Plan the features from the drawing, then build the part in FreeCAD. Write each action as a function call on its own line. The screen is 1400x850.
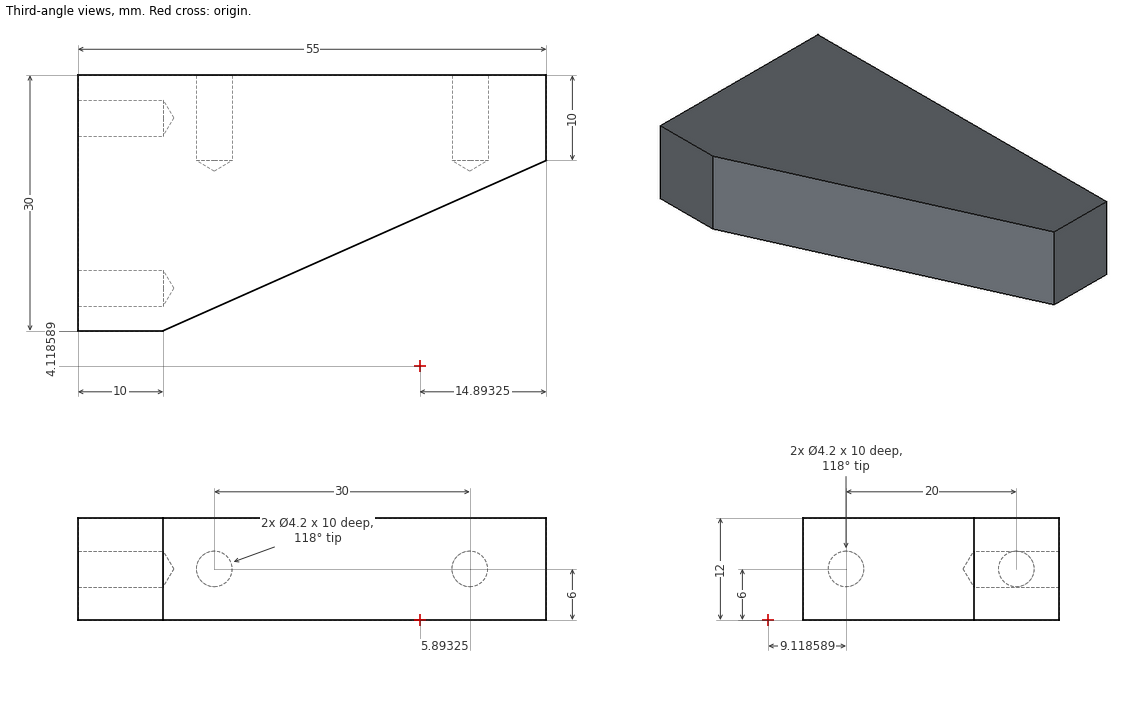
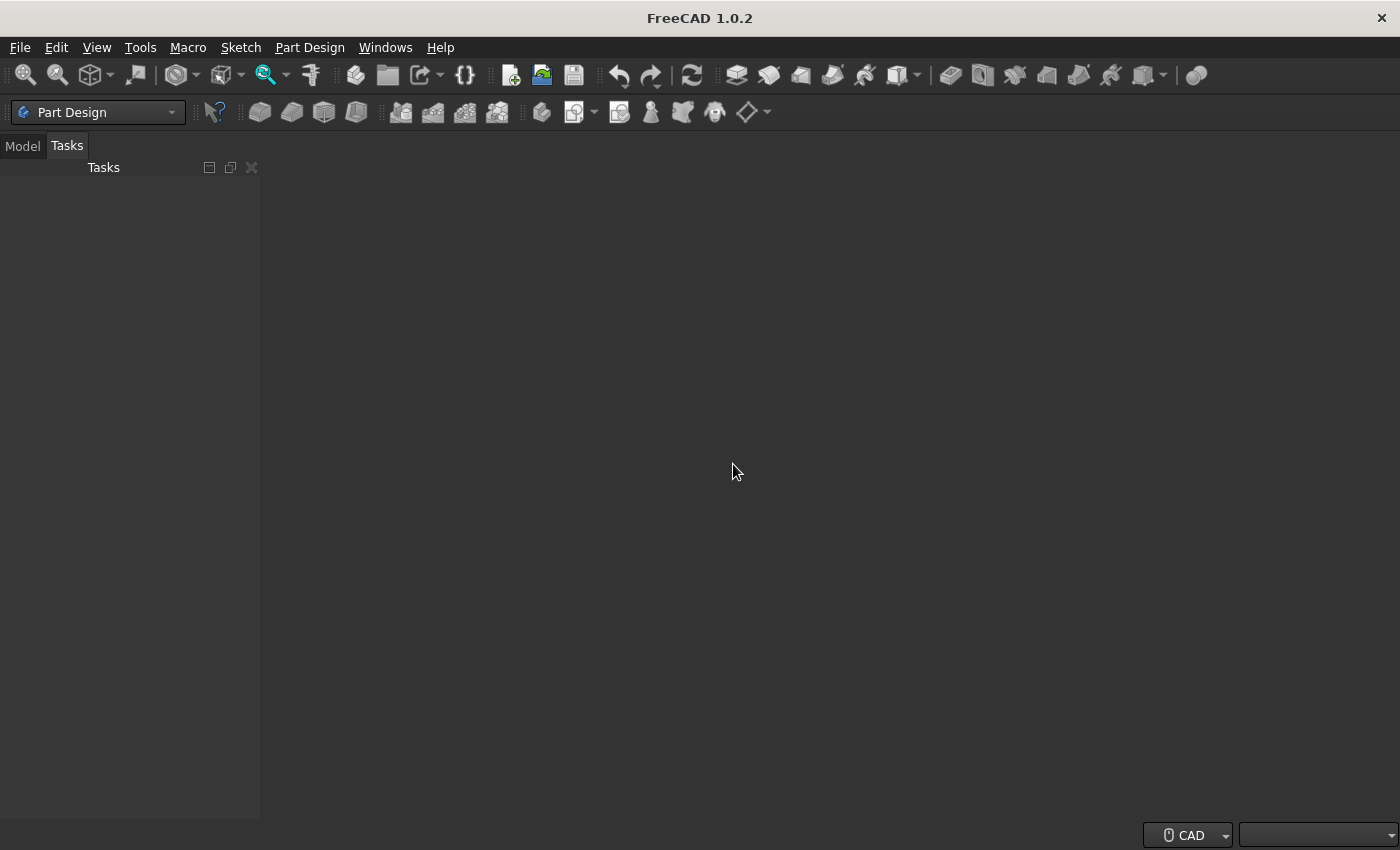
click(510, 76)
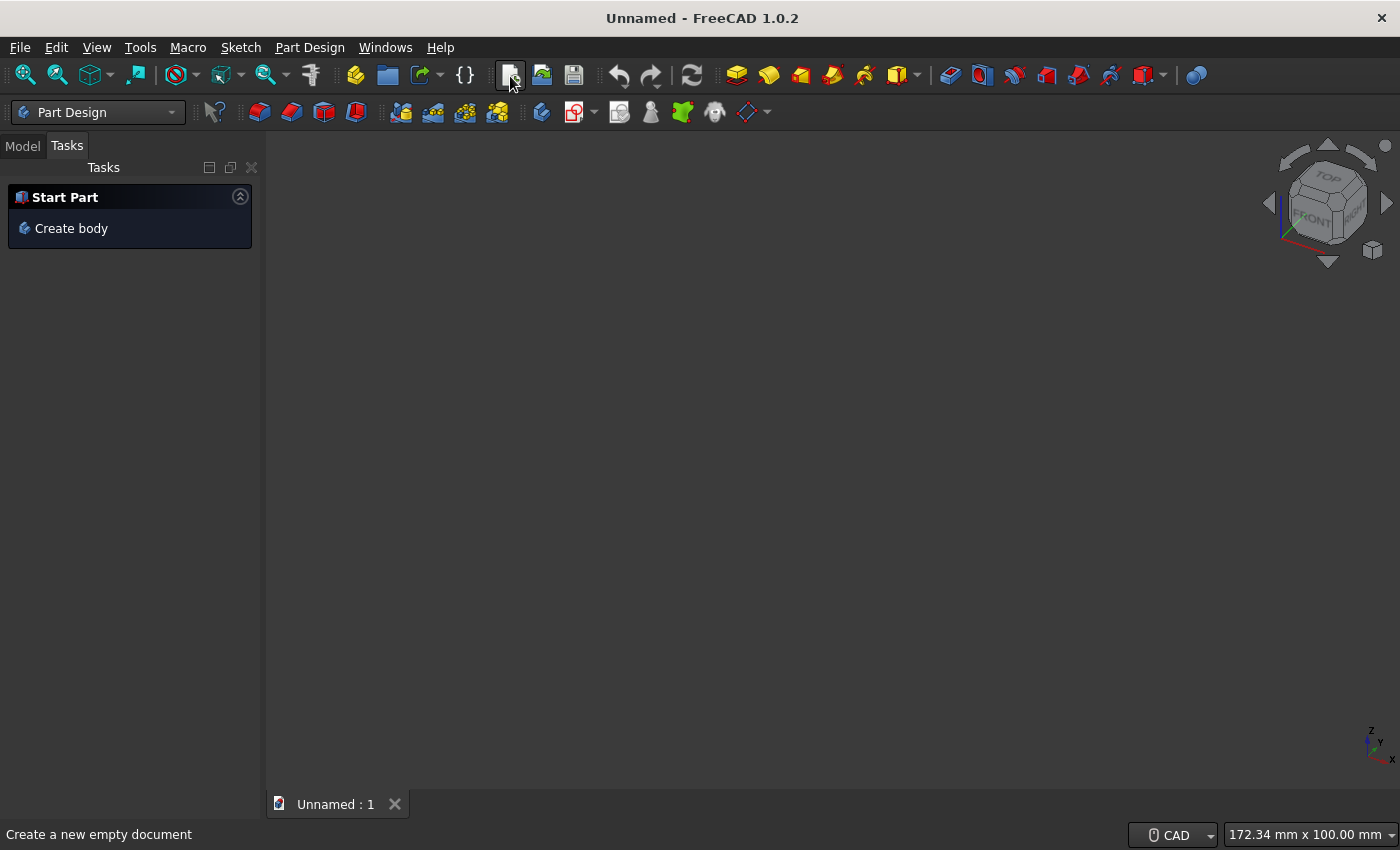
click(574, 112)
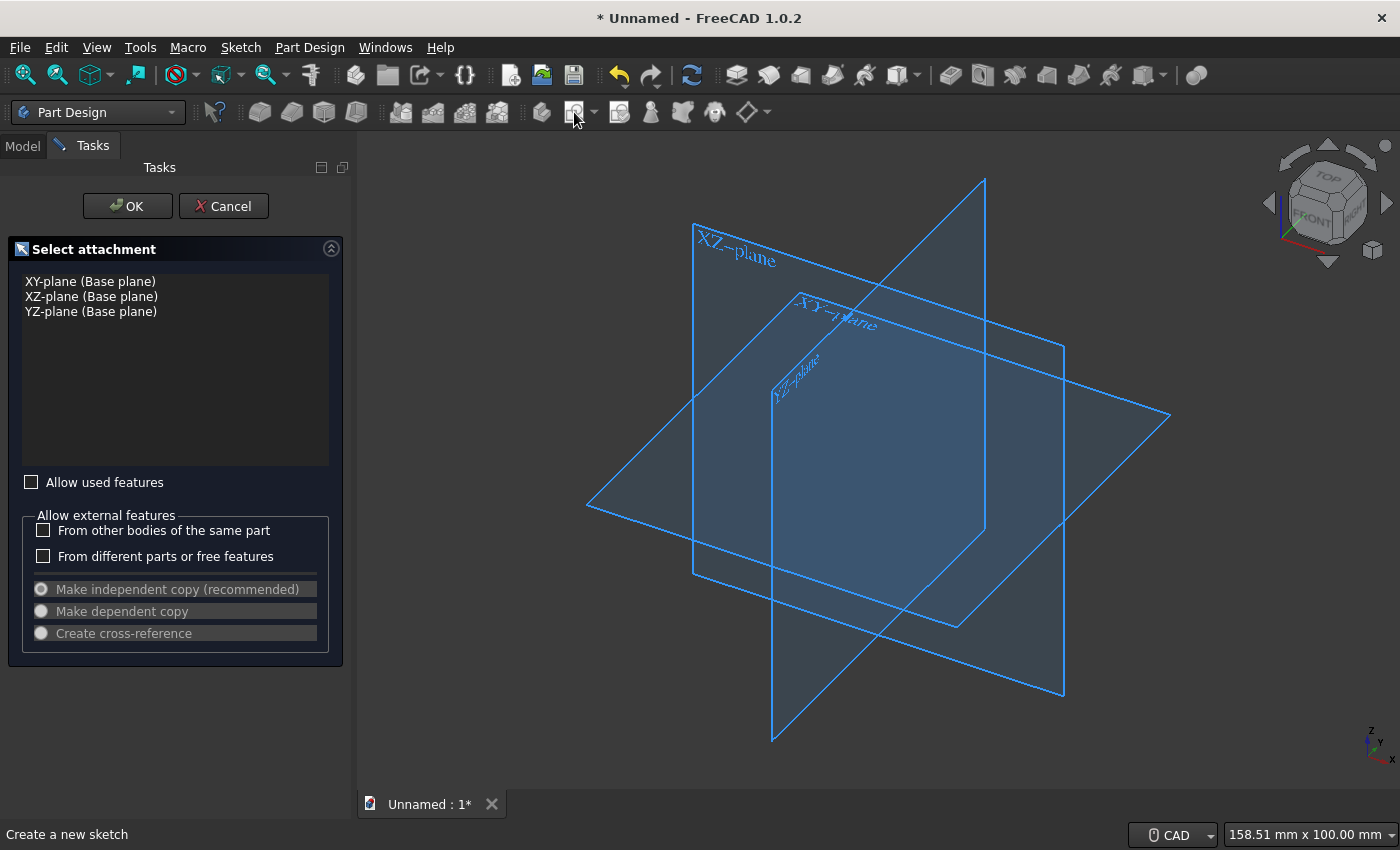
click(82, 282)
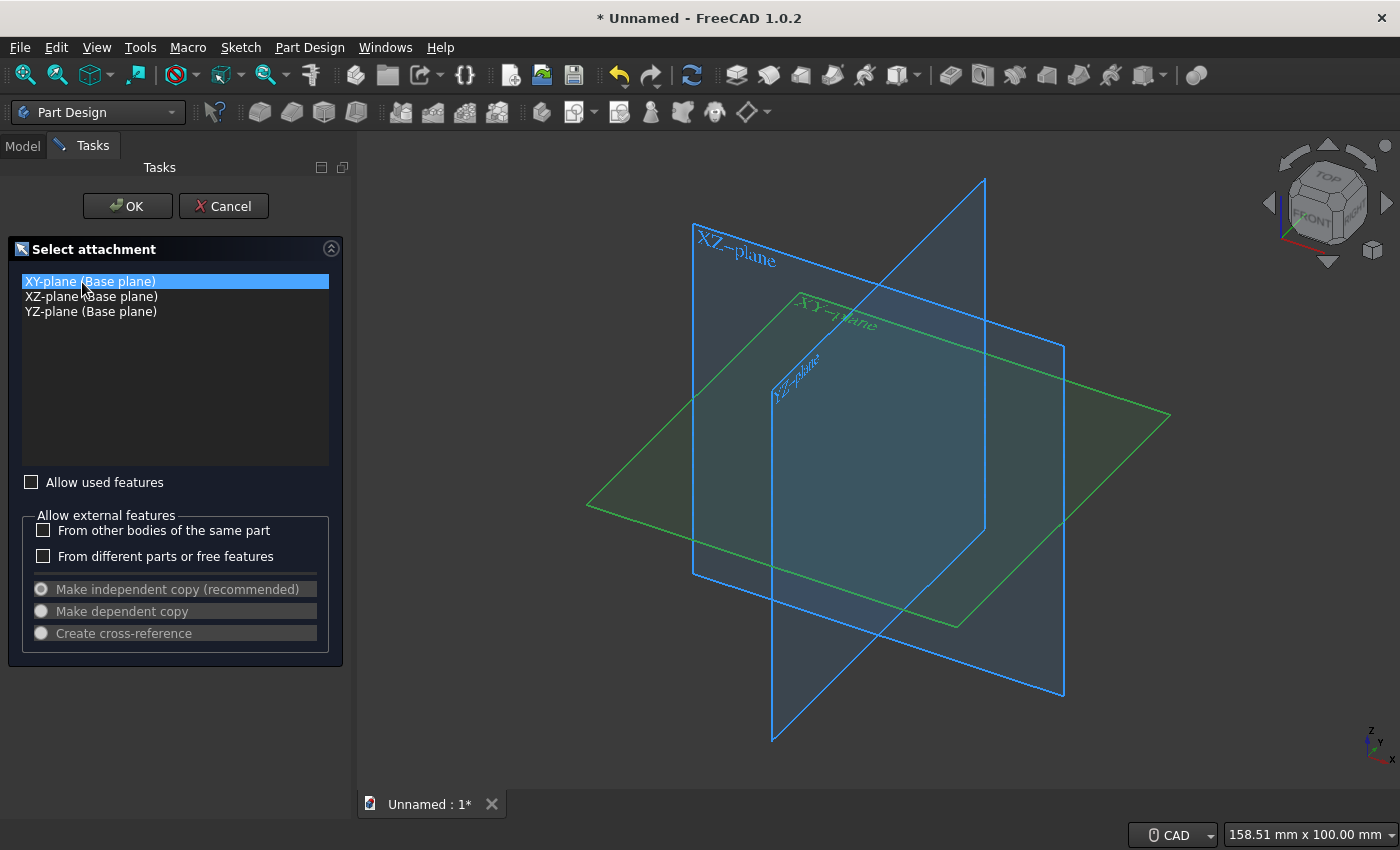
click(128, 206)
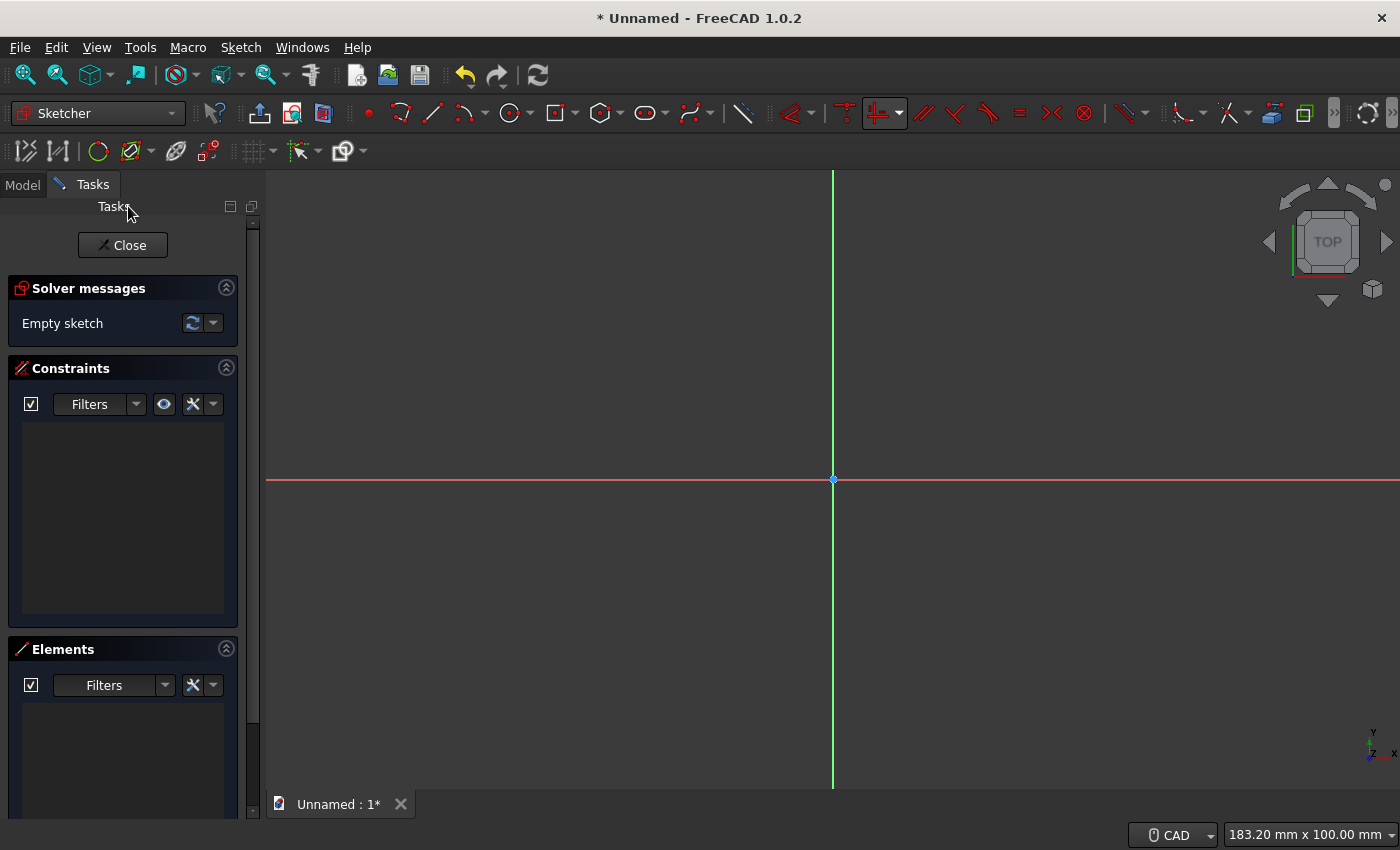
scroll(743, 245, up, 3)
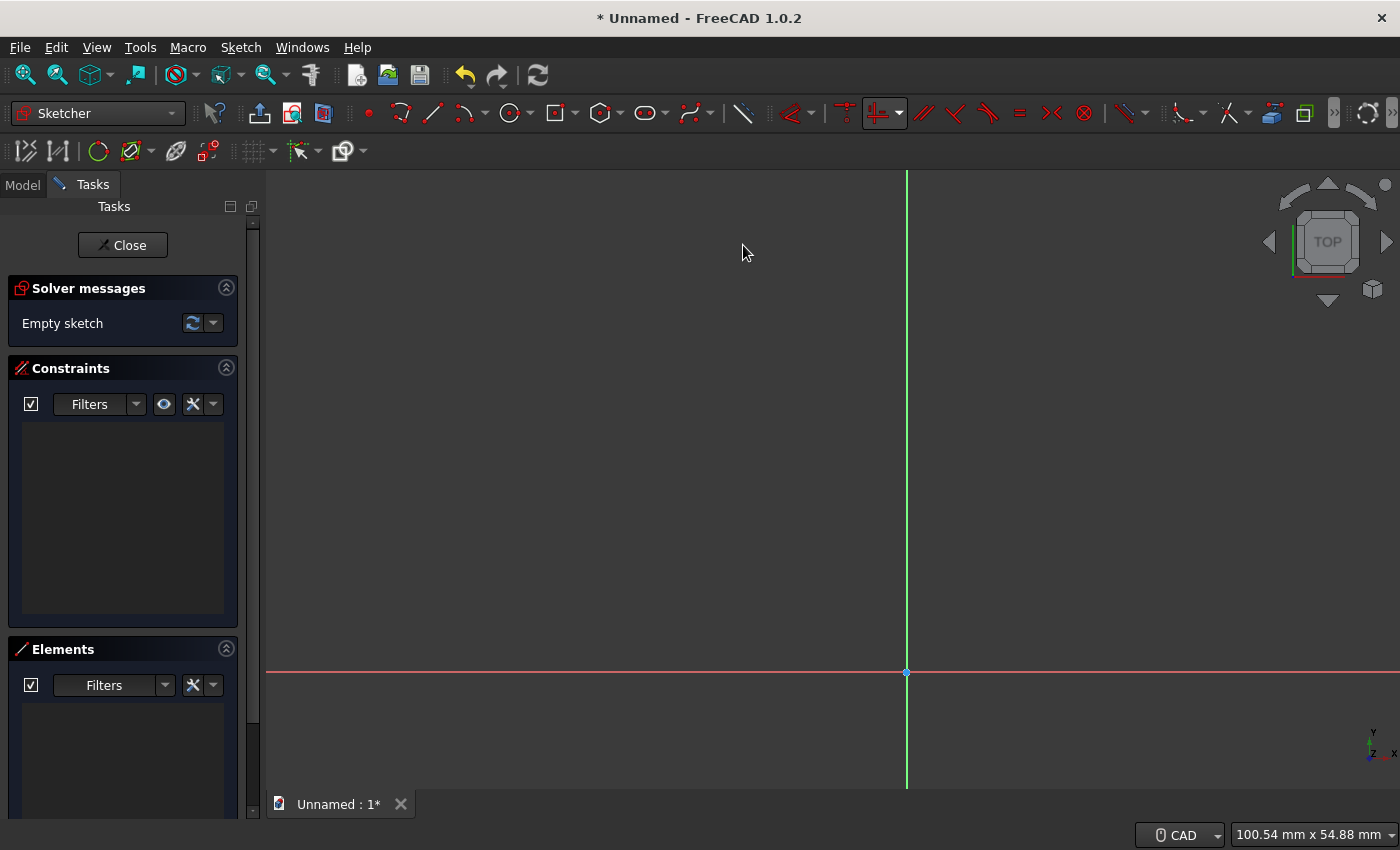
click(402, 114)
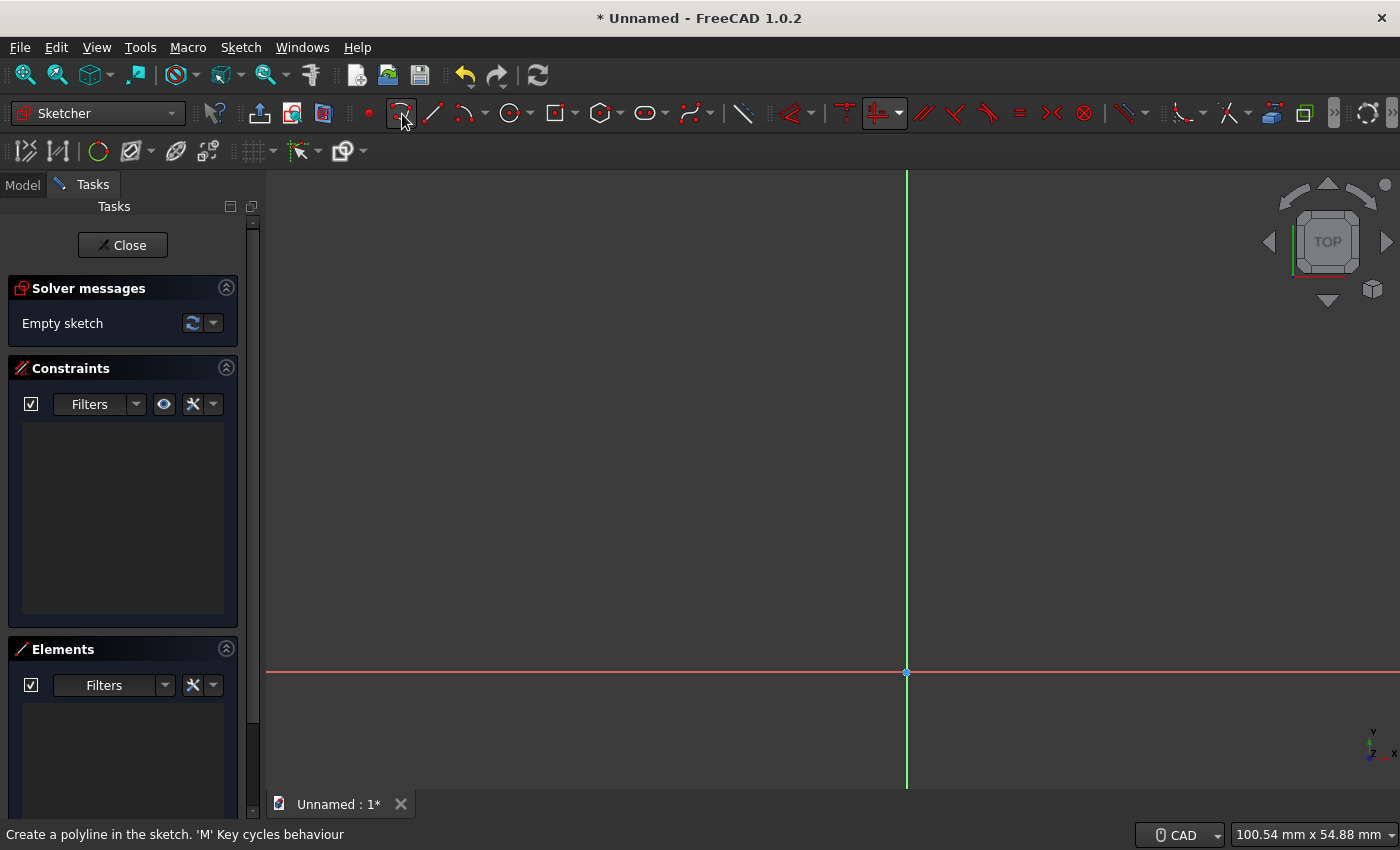
click(1075, 400)
click(1075, 287)
click(454, 287)
click(454, 626)
click(567, 626)
click(1075, 401)
key(Escape)
key(Escape)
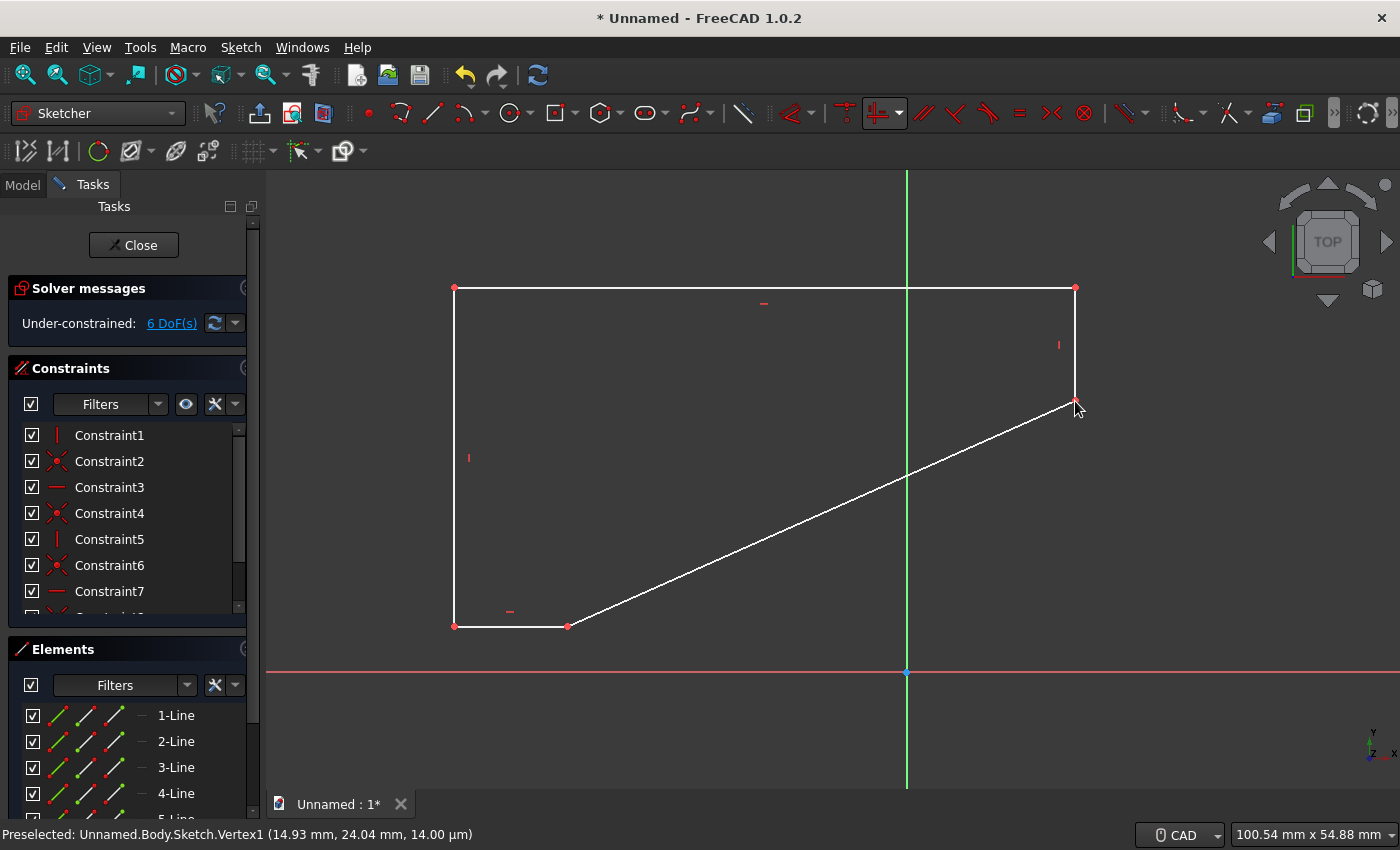
click(1075, 367)